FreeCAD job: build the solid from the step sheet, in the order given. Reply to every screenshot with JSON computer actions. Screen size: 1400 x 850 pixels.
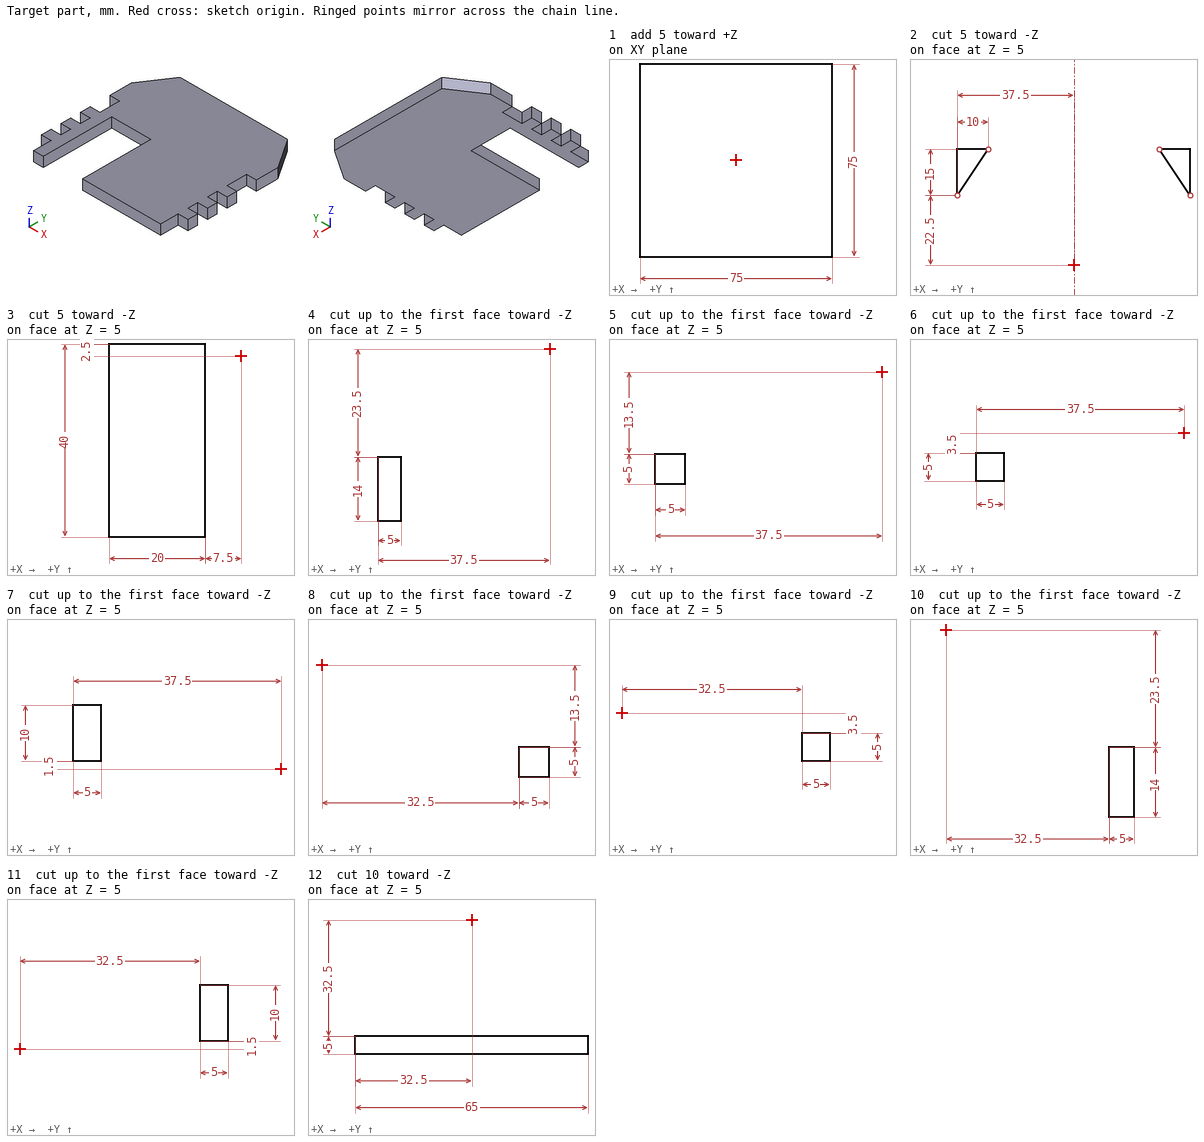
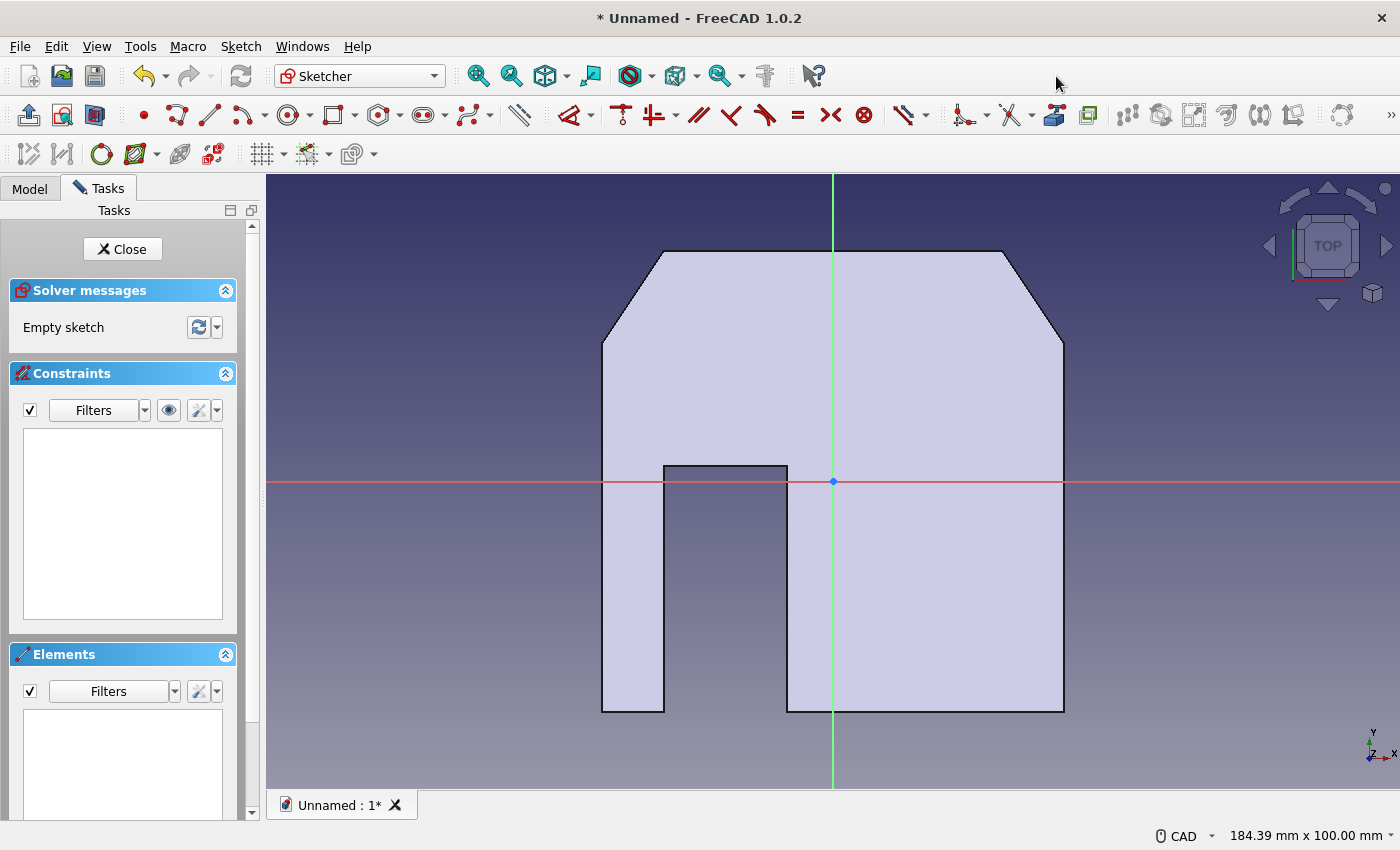
{"action": "scroll", "coordinate": [581, 717], "scroll_direction": "up", "scroll_amount": 8}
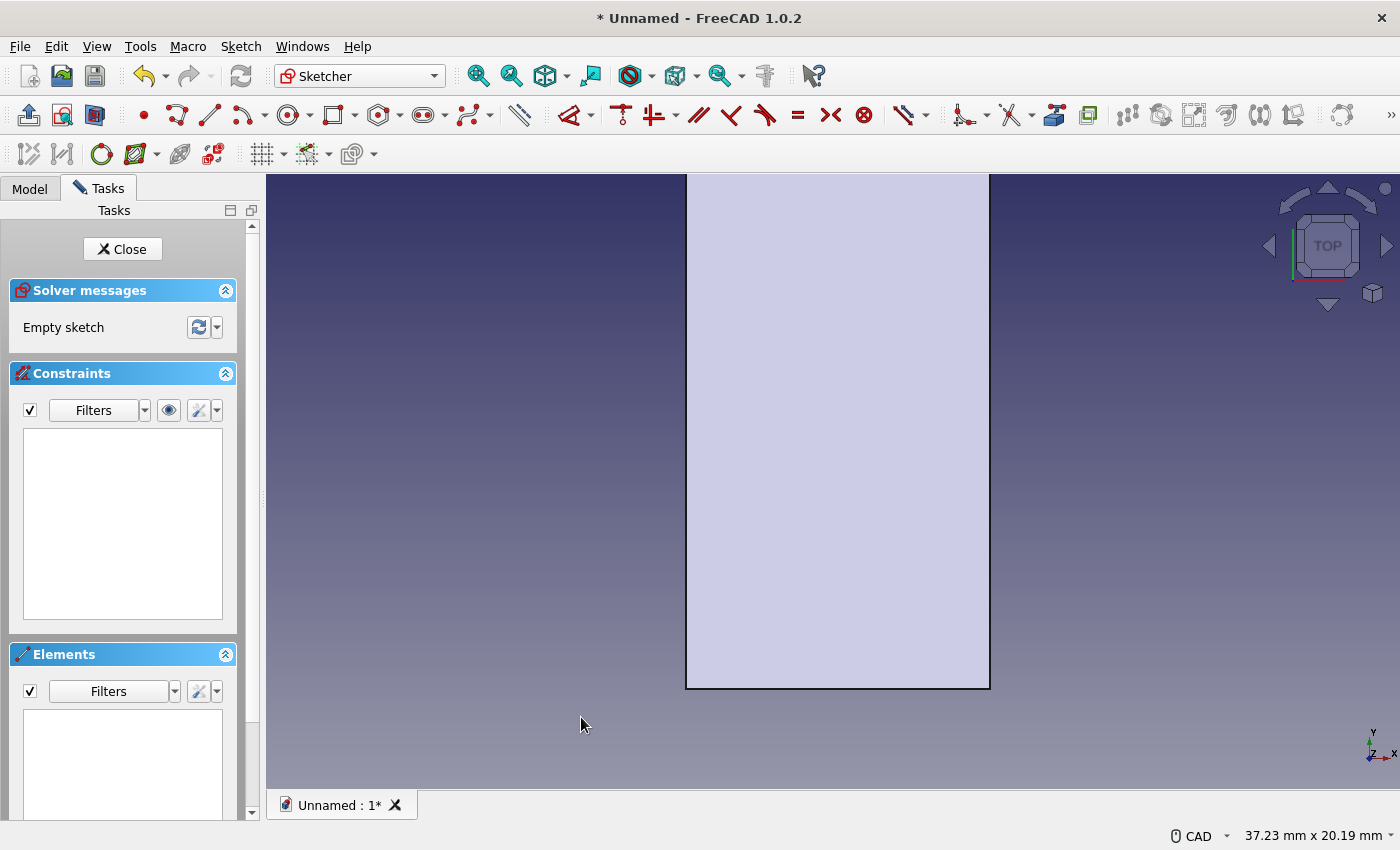
{"action": "left_click", "coordinate": [332, 116]}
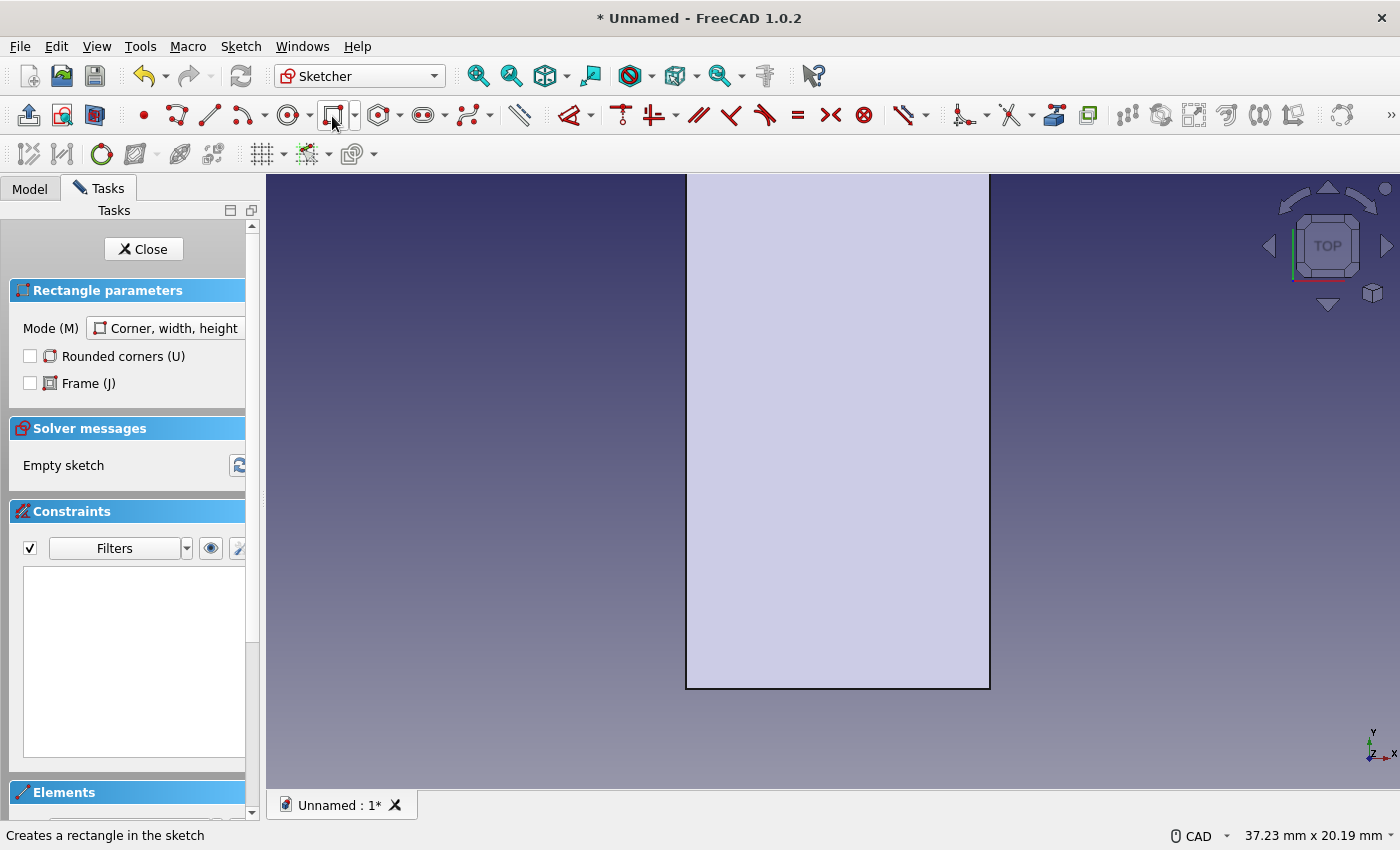
{"action": "left_click", "coordinate": [686, 263]}
{"action": "left_click", "coordinate": [838, 689]}
{"action": "key", "text": "Escape"}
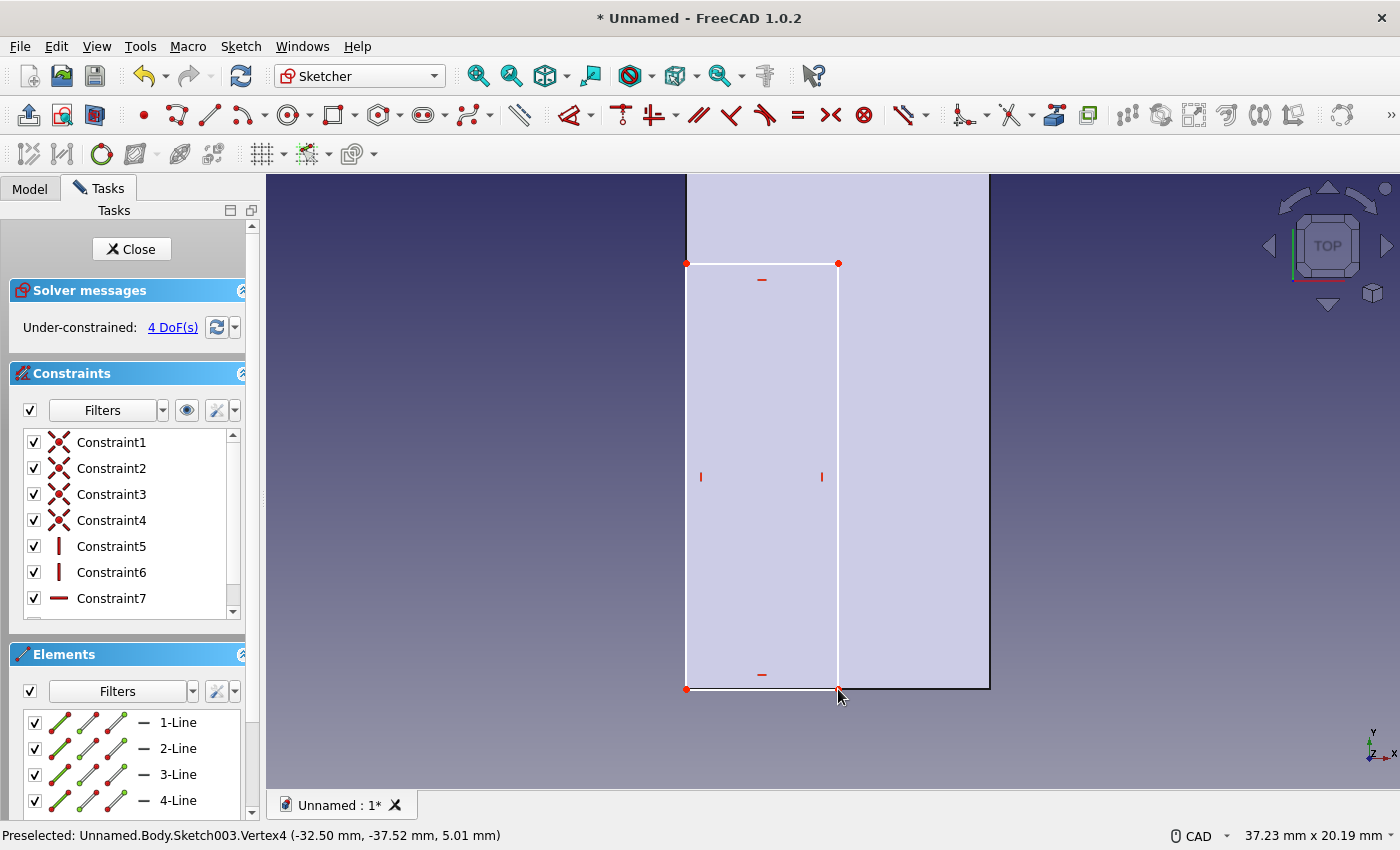
{"action": "left_click", "coordinate": [568, 116]}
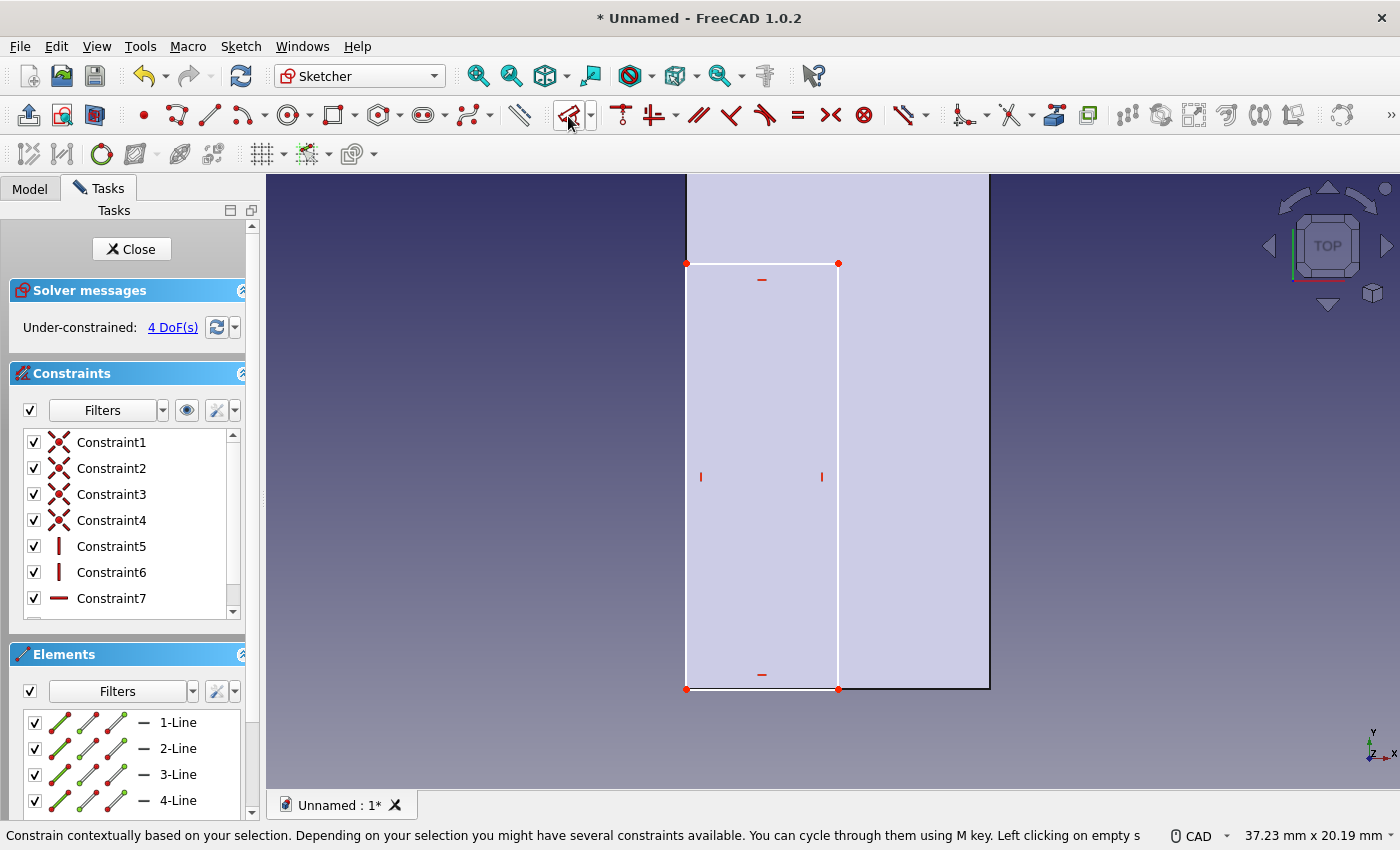
{"action": "left_click", "coordinate": [732, 690]}
{"action": "left_click", "coordinate": [762, 724]}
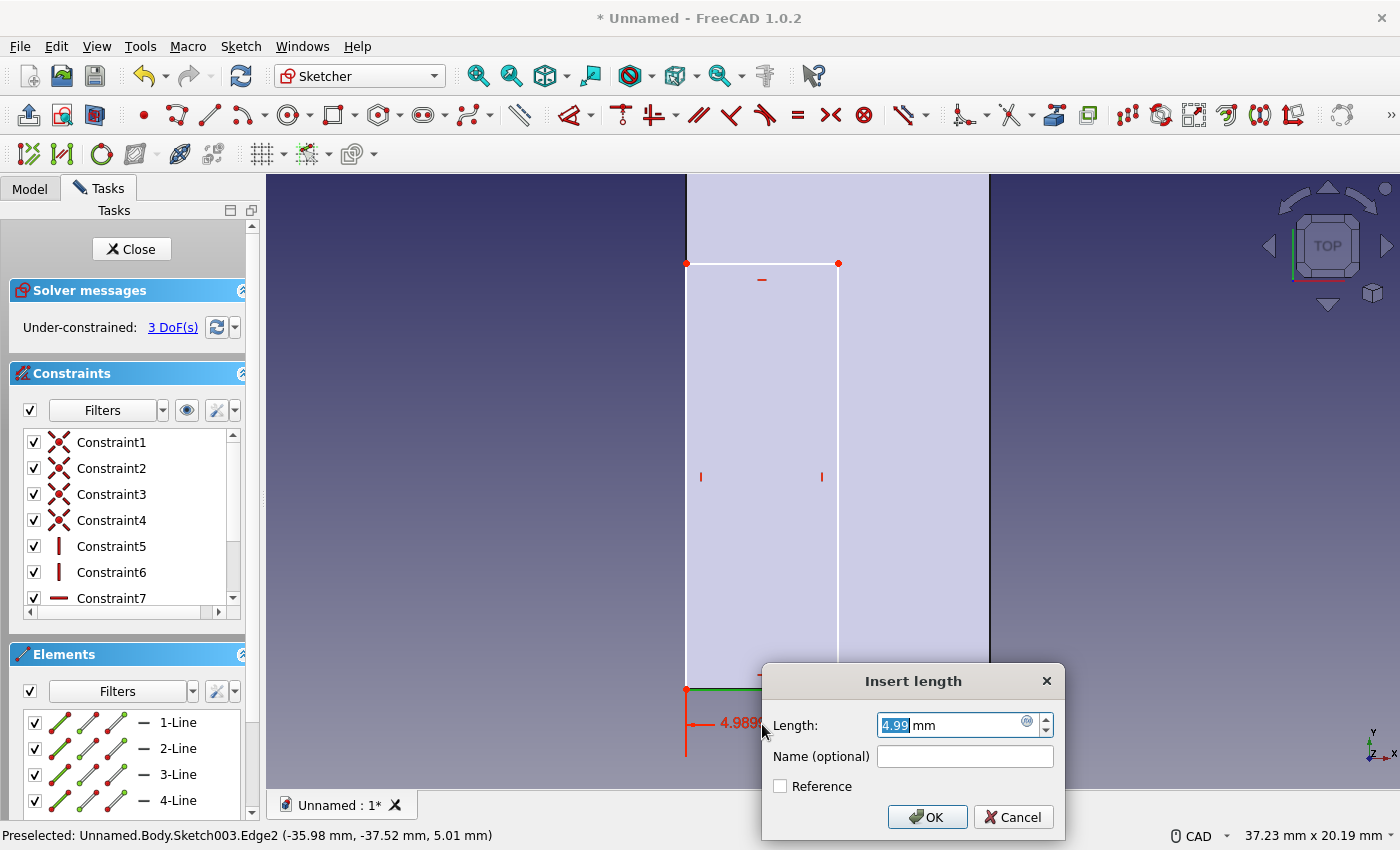
{"action": "type", "text": "5"}
{"action": "key", "text": "Return"}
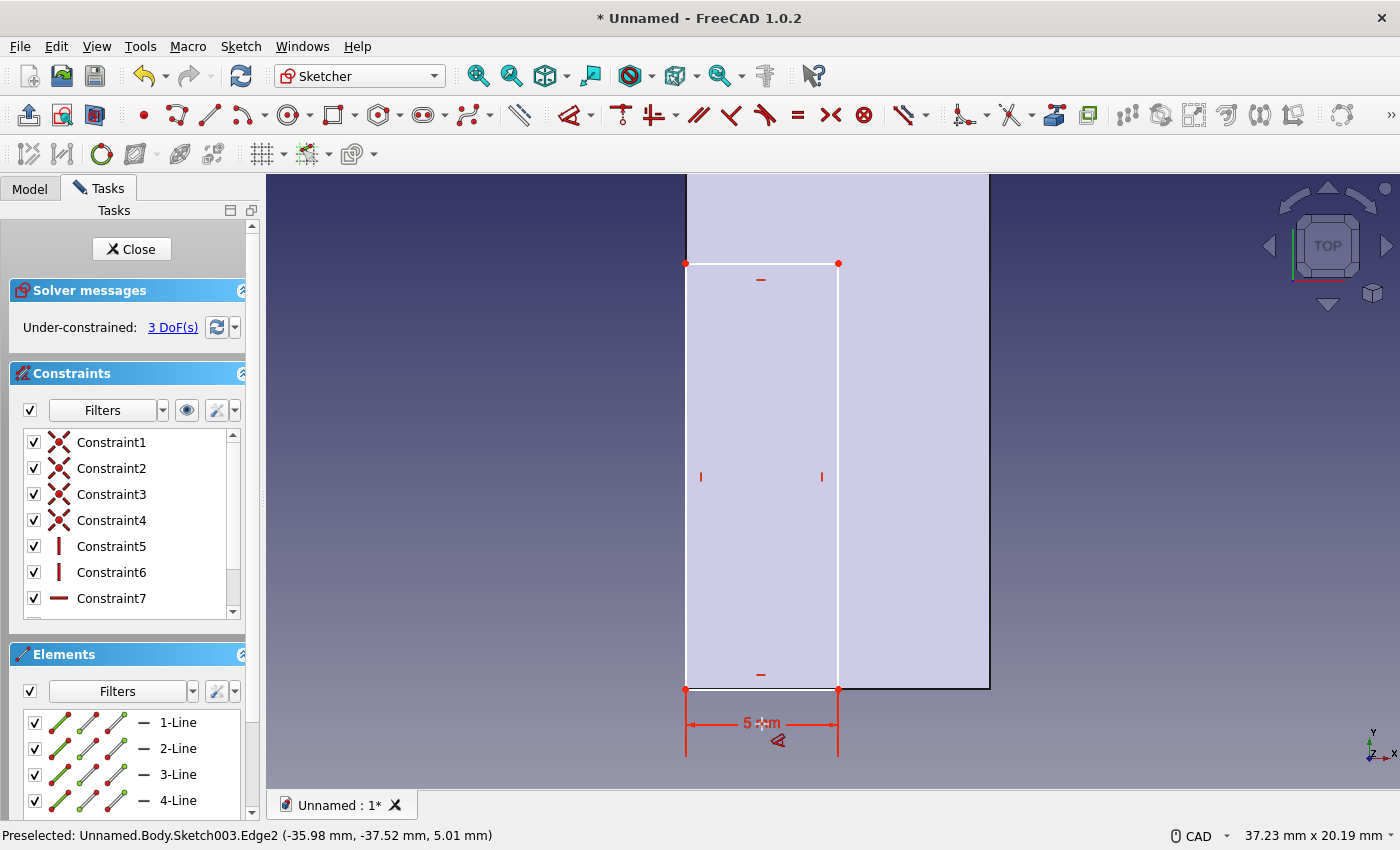
{"action": "left_click", "coordinate": [686, 392]}
{"action": "left_click", "coordinate": [652, 477]}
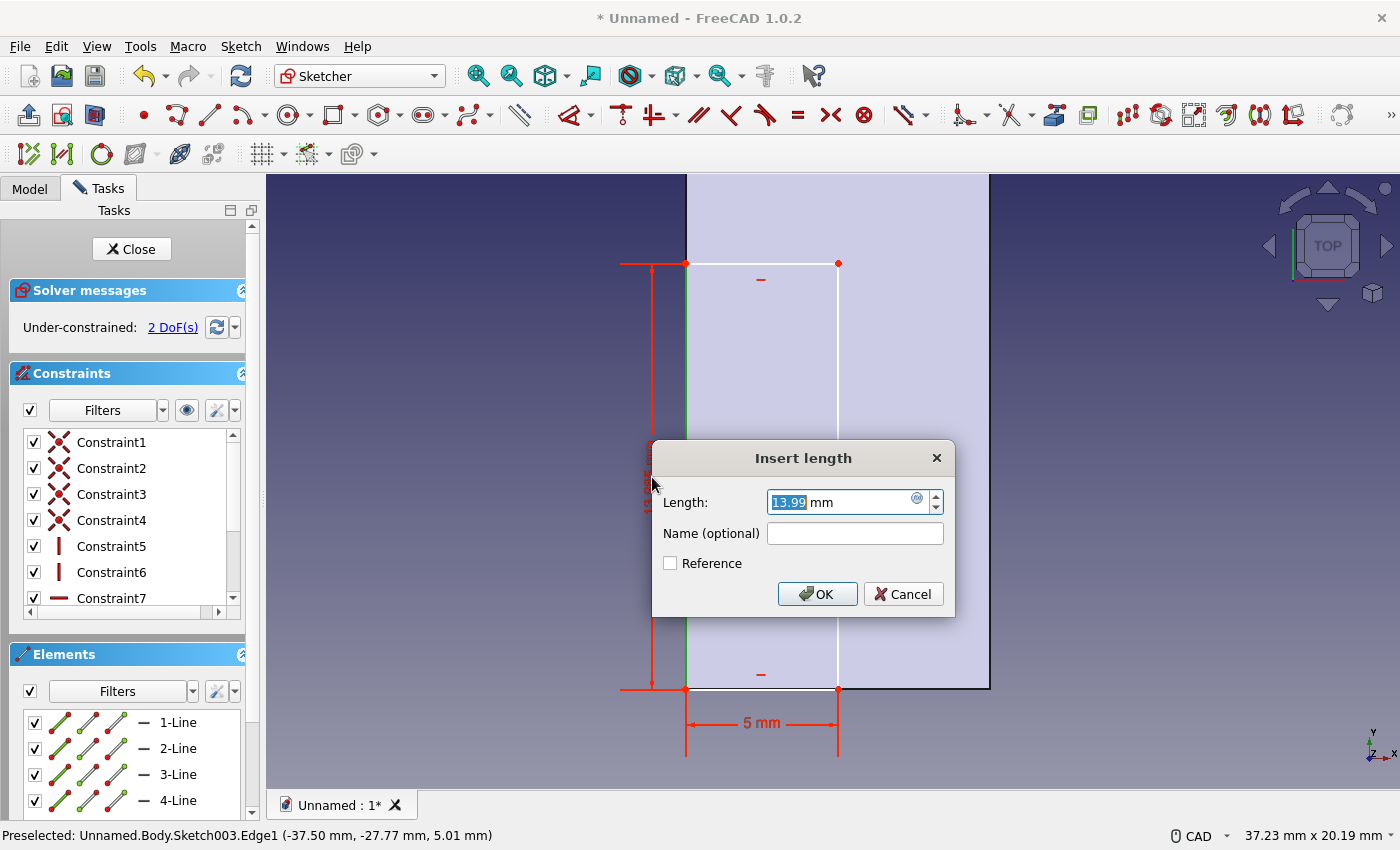
{"action": "type", "text": "14"}
{"action": "key", "text": "Return"}